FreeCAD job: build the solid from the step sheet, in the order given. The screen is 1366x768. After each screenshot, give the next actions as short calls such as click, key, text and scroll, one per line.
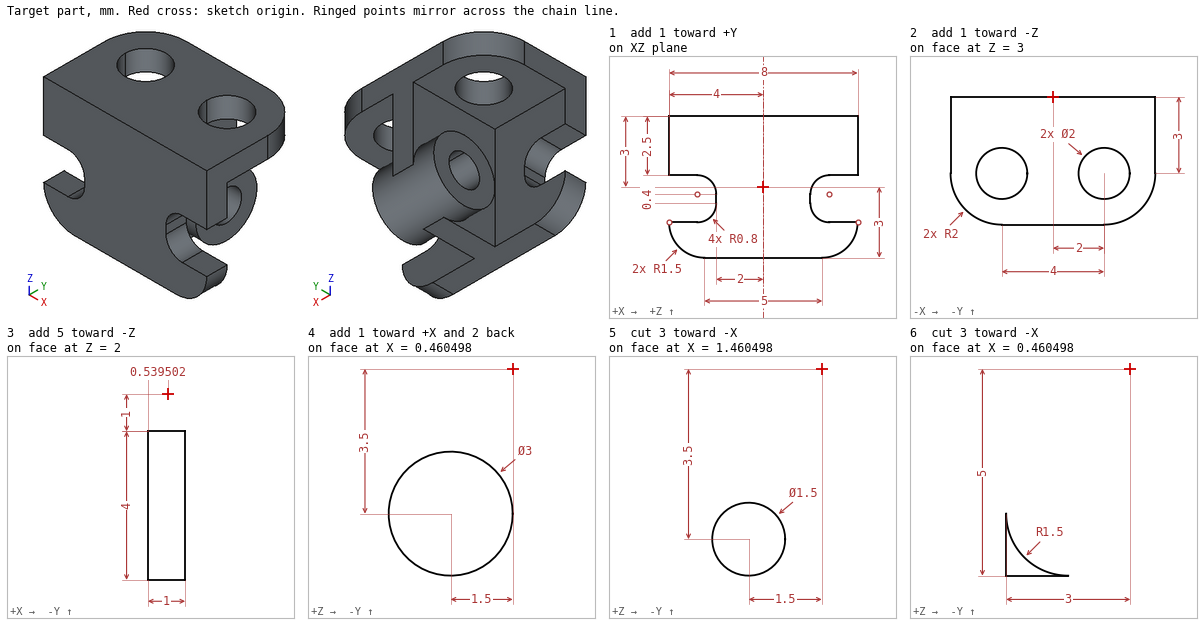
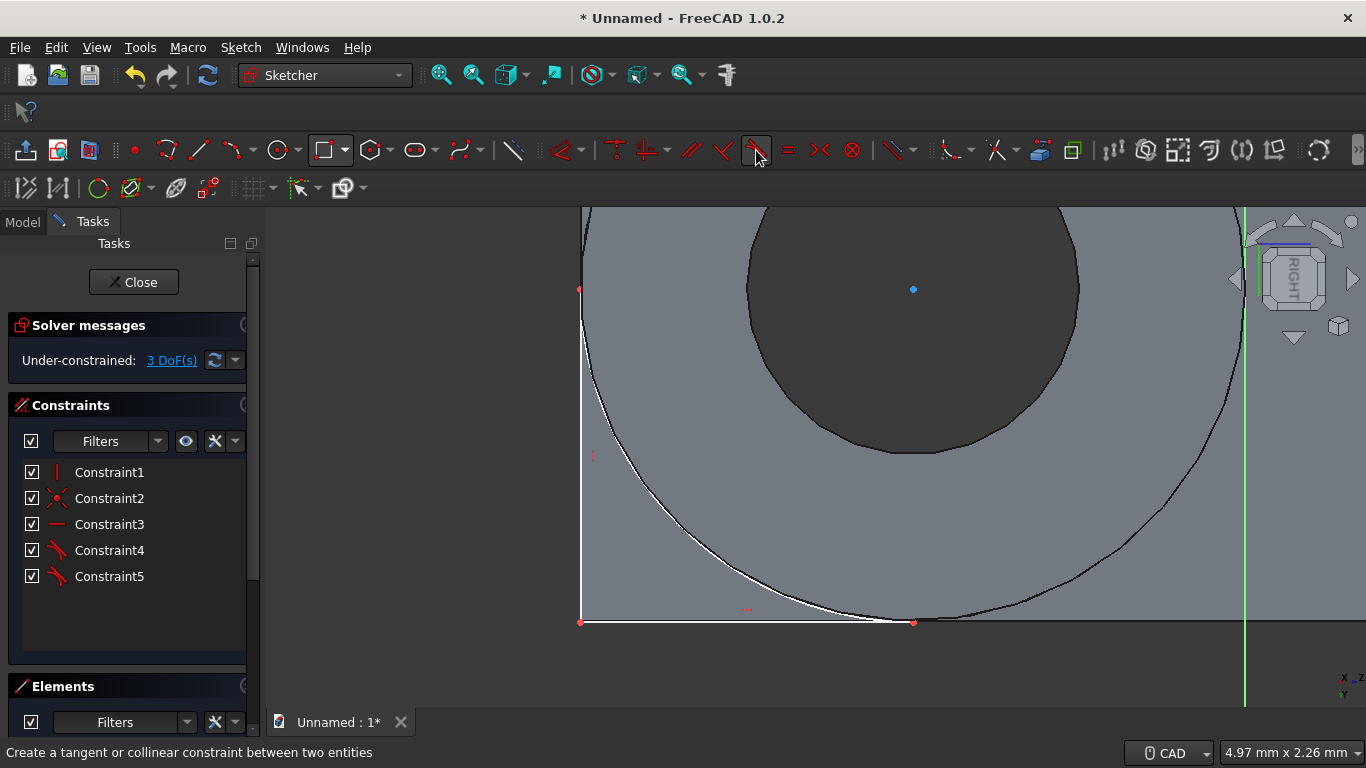
click(560, 150)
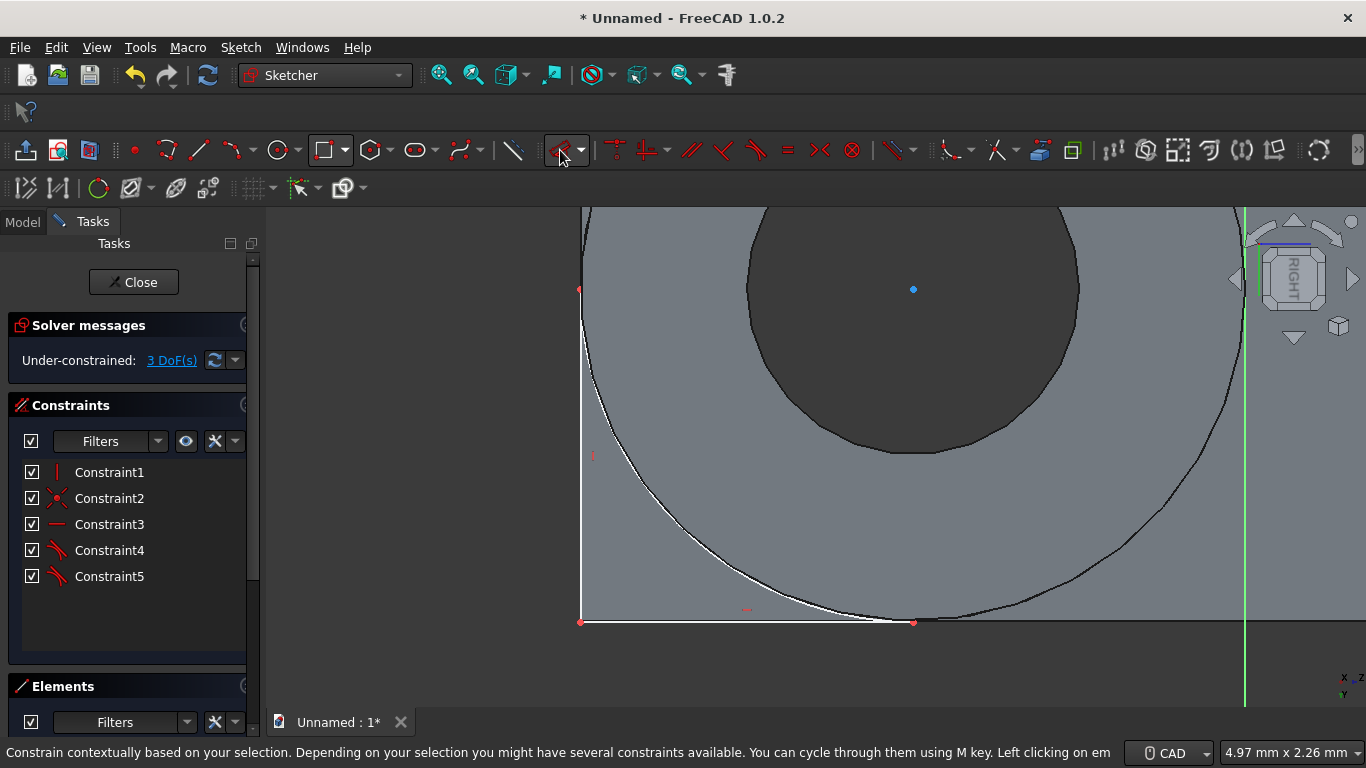
click(617, 440)
click(549, 278)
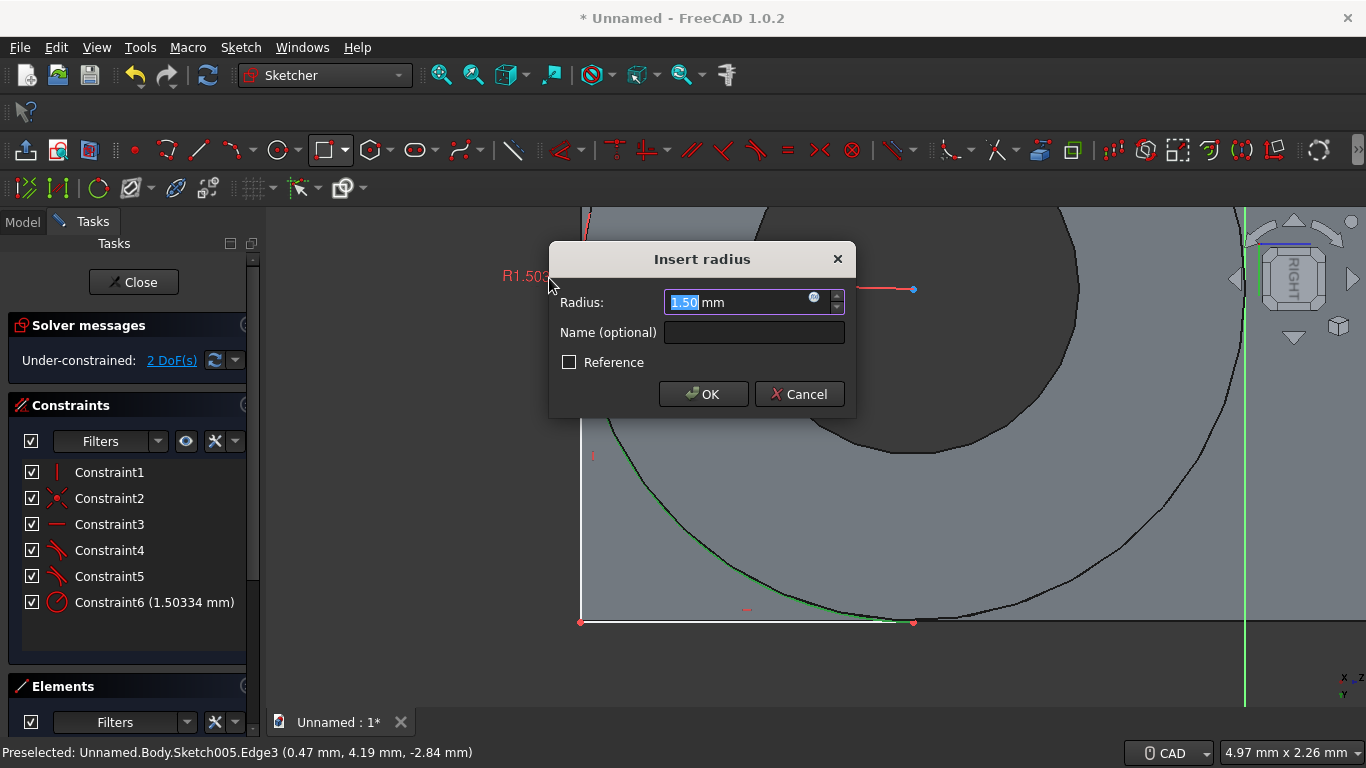
text(1.5)
key(Return)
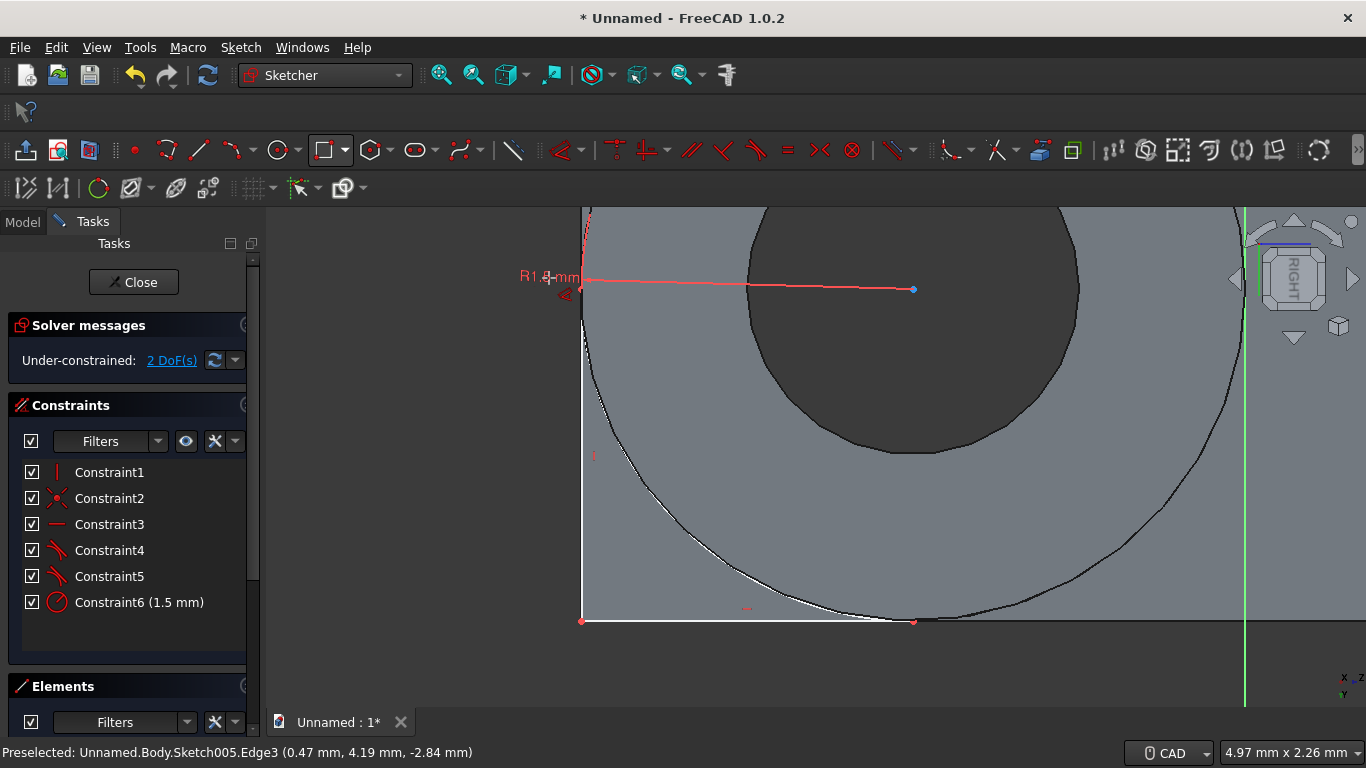
click(582, 289)
click(891, 323)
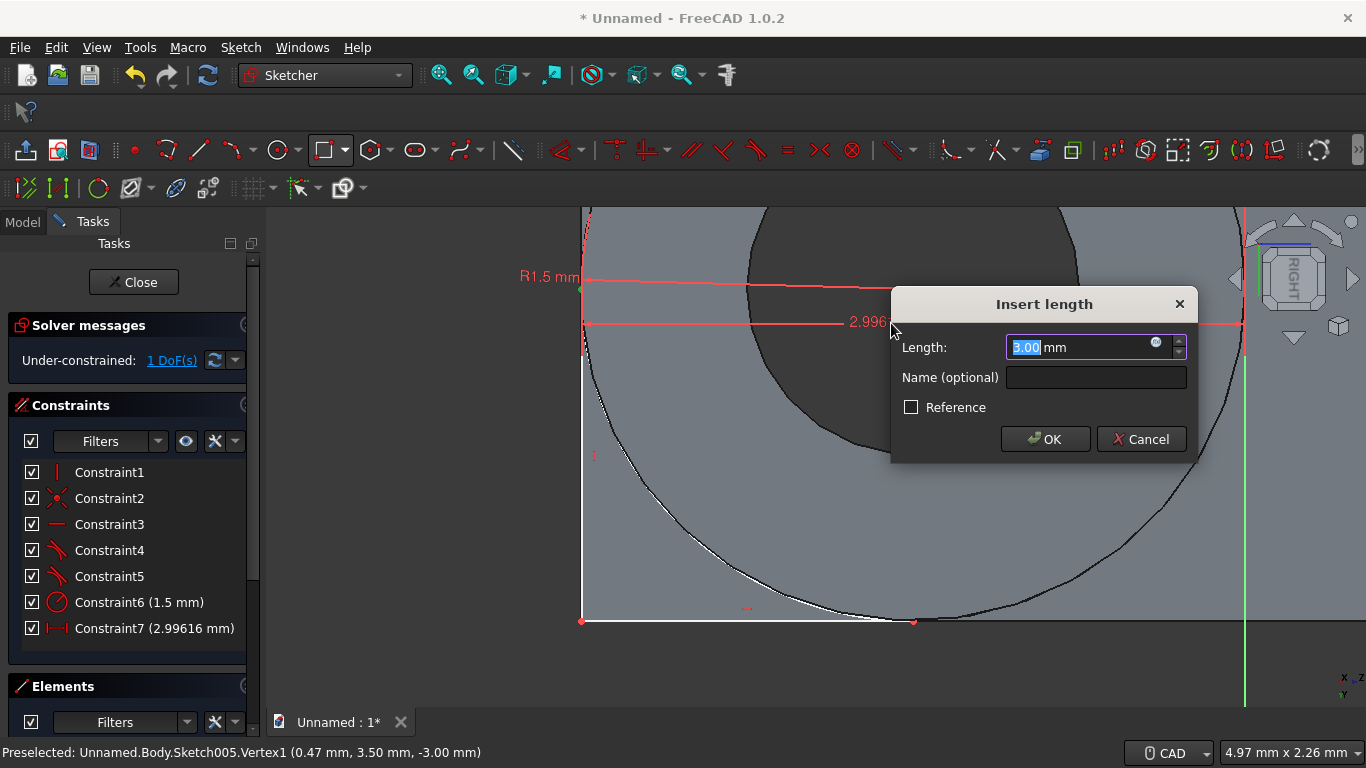
text(3)
key(Return)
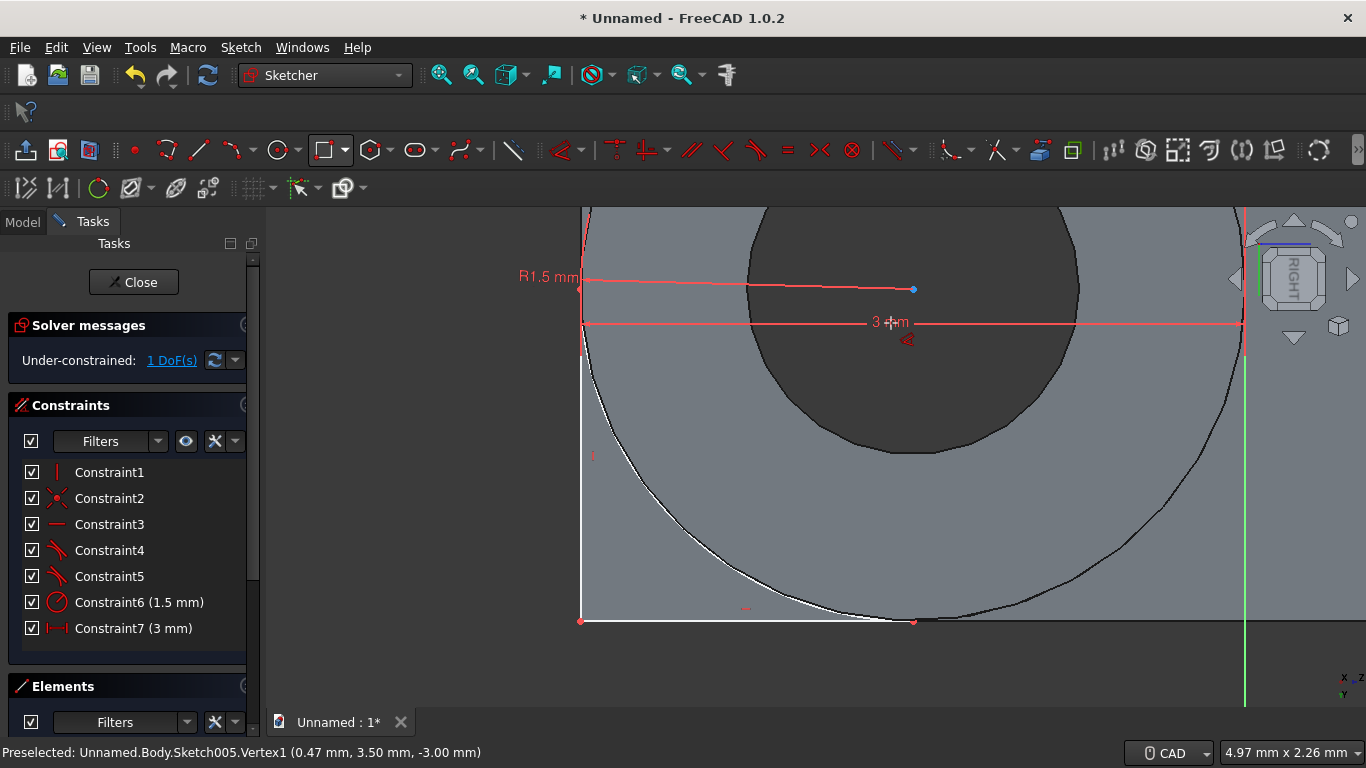
click(581, 621)
click(547, 428)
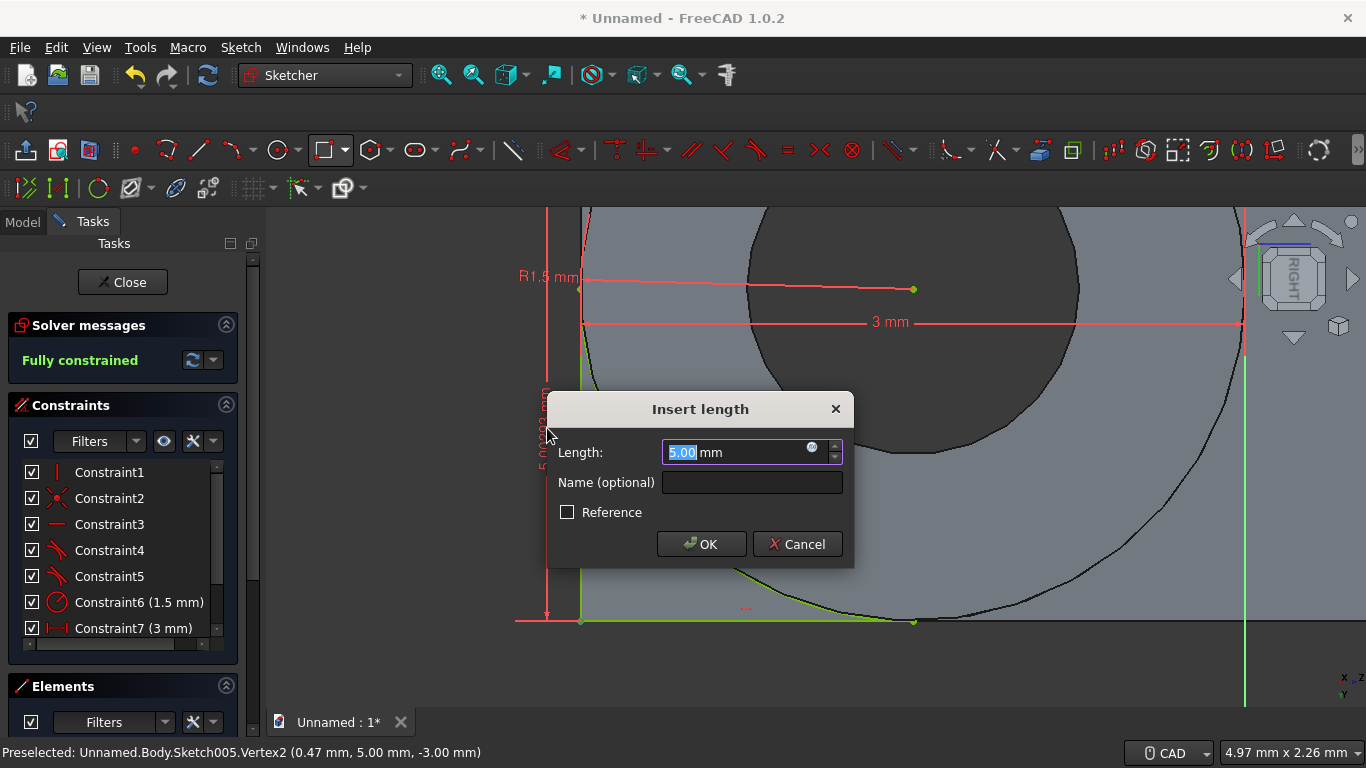
text(5)
key(Return)
key(Escape)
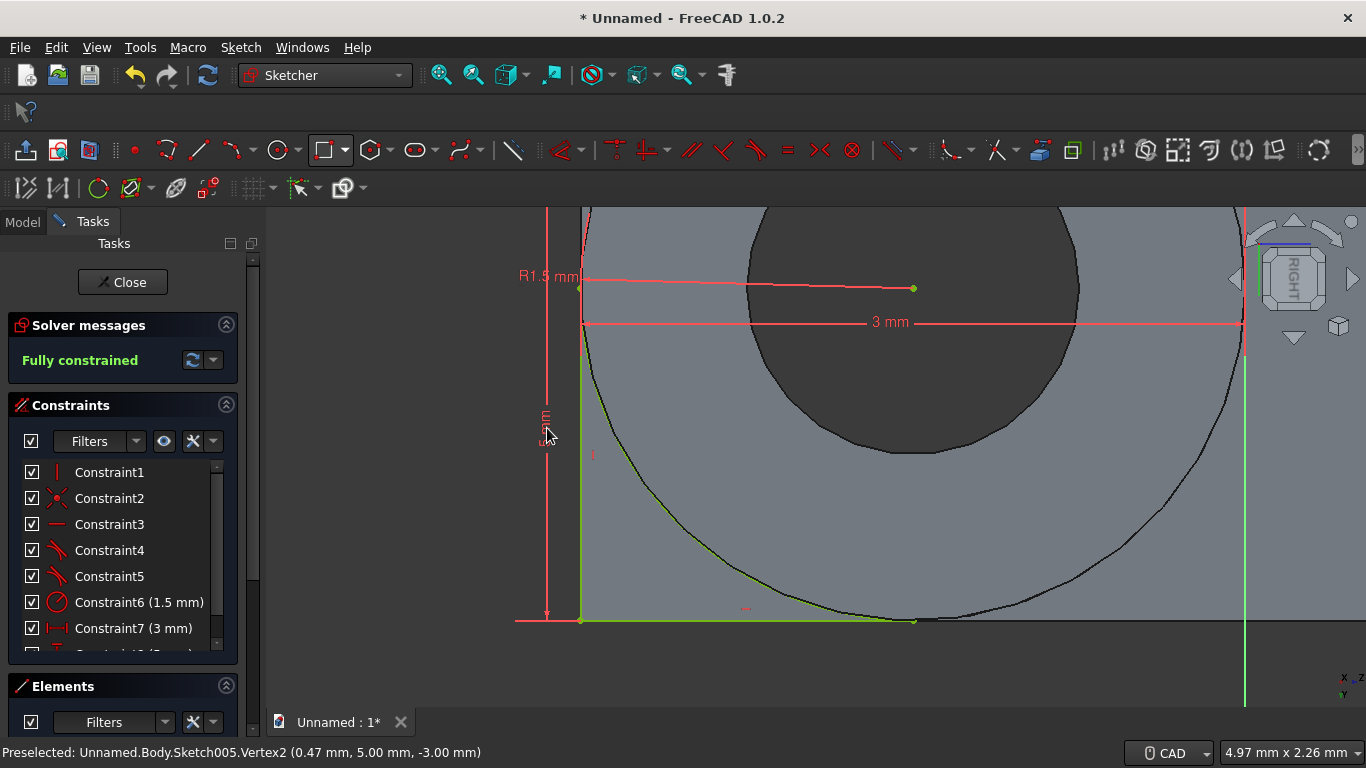
click(123, 282)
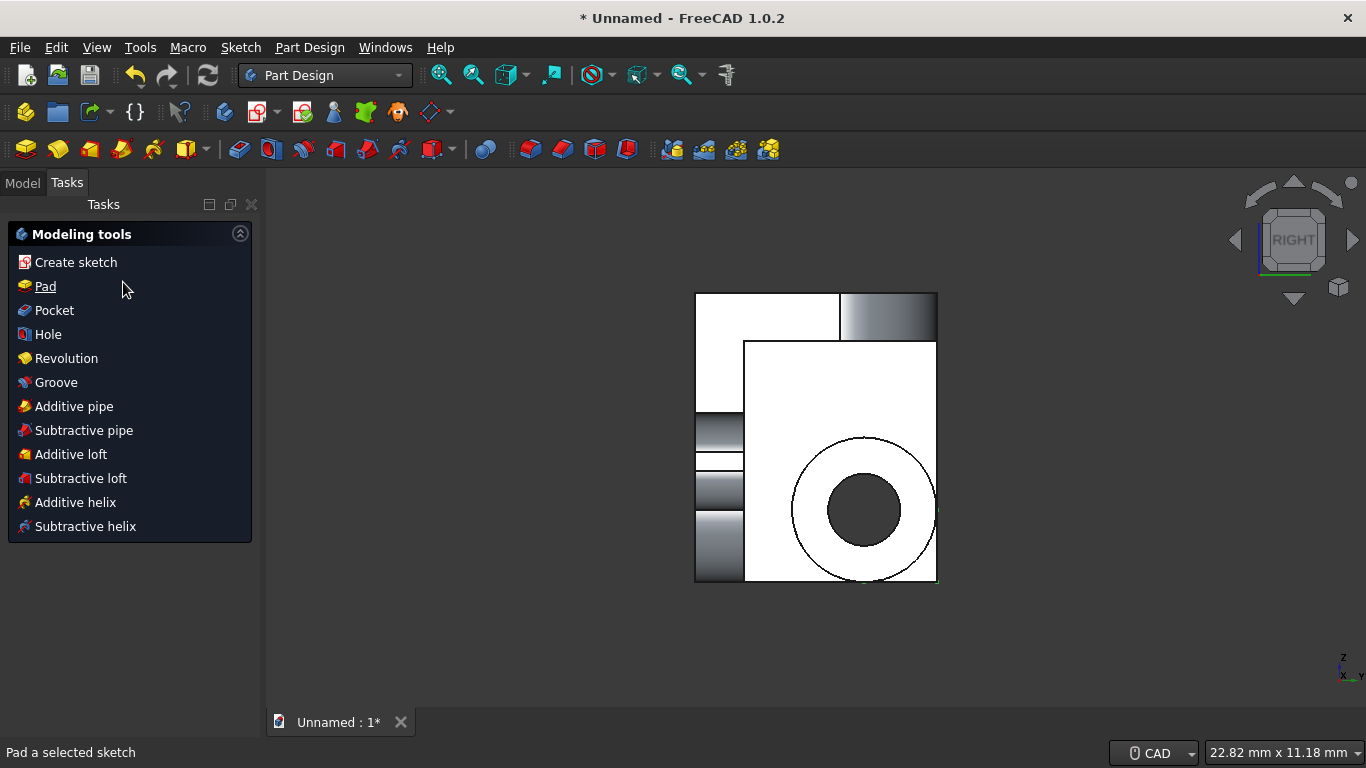
click(240, 150)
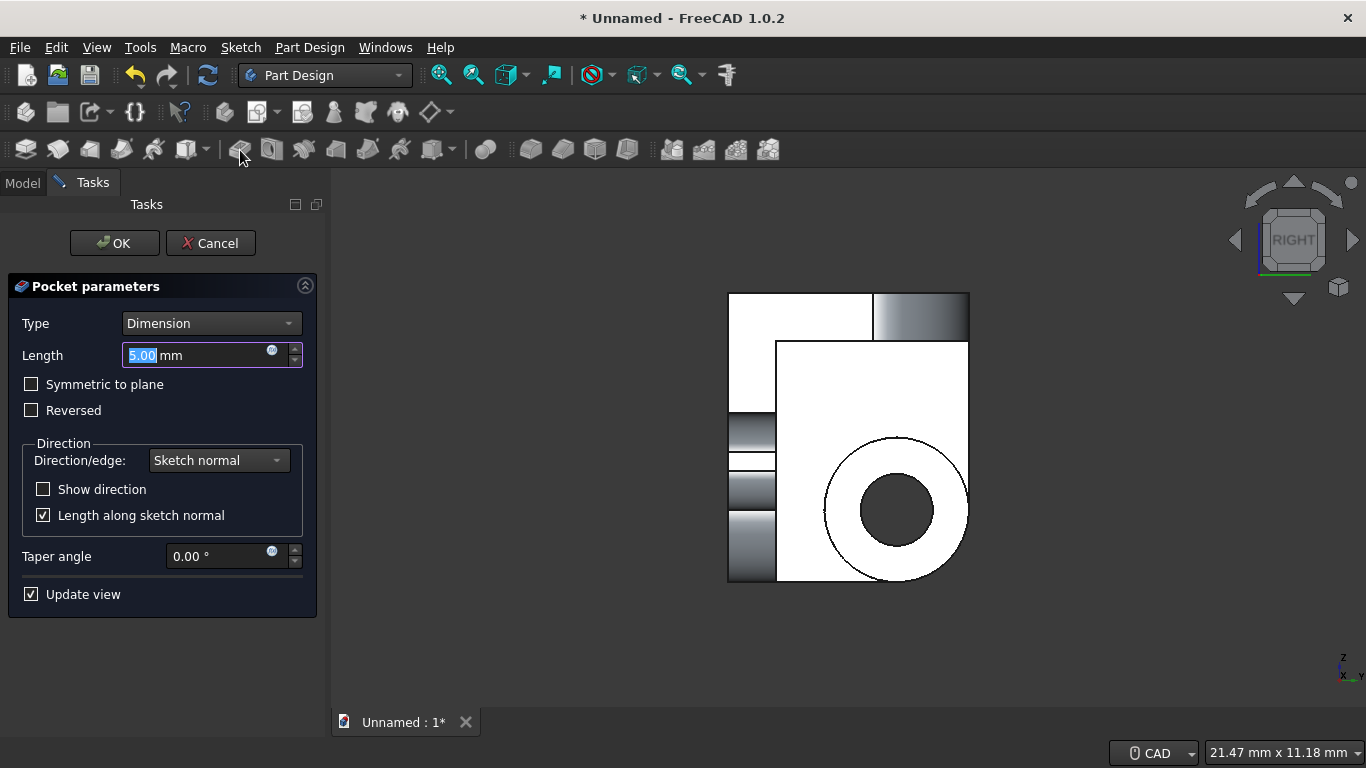
text(3)
key(Tab)